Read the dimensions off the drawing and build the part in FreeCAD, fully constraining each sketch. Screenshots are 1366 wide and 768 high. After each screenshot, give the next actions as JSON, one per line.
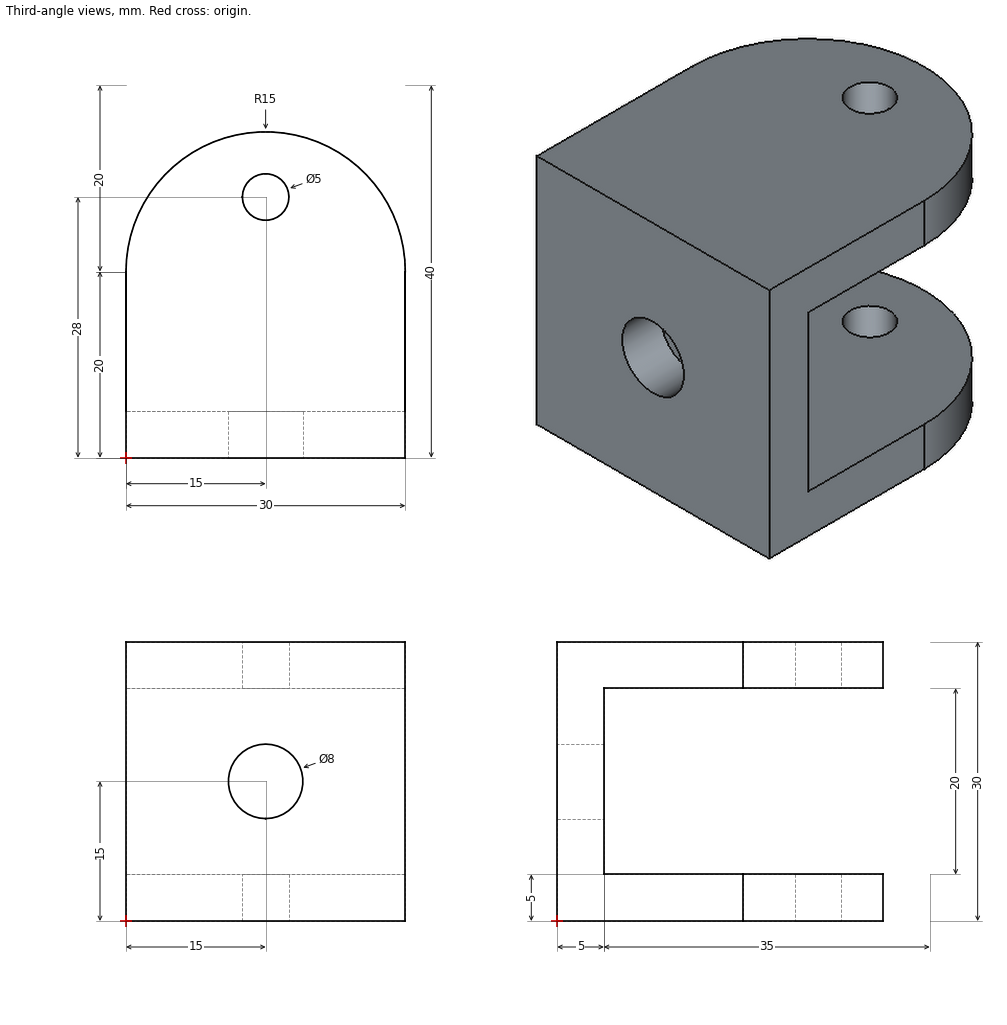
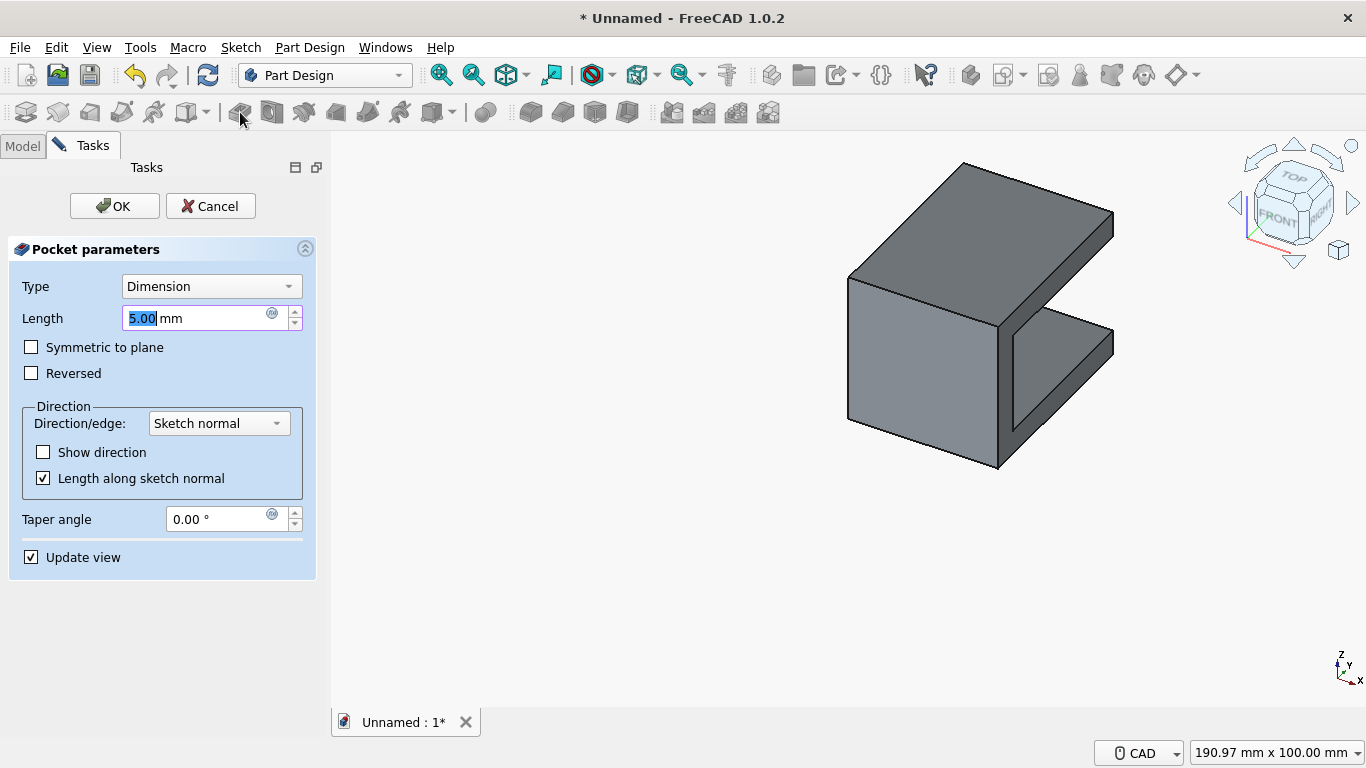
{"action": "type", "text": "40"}
{"action": "key", "text": "Tab"}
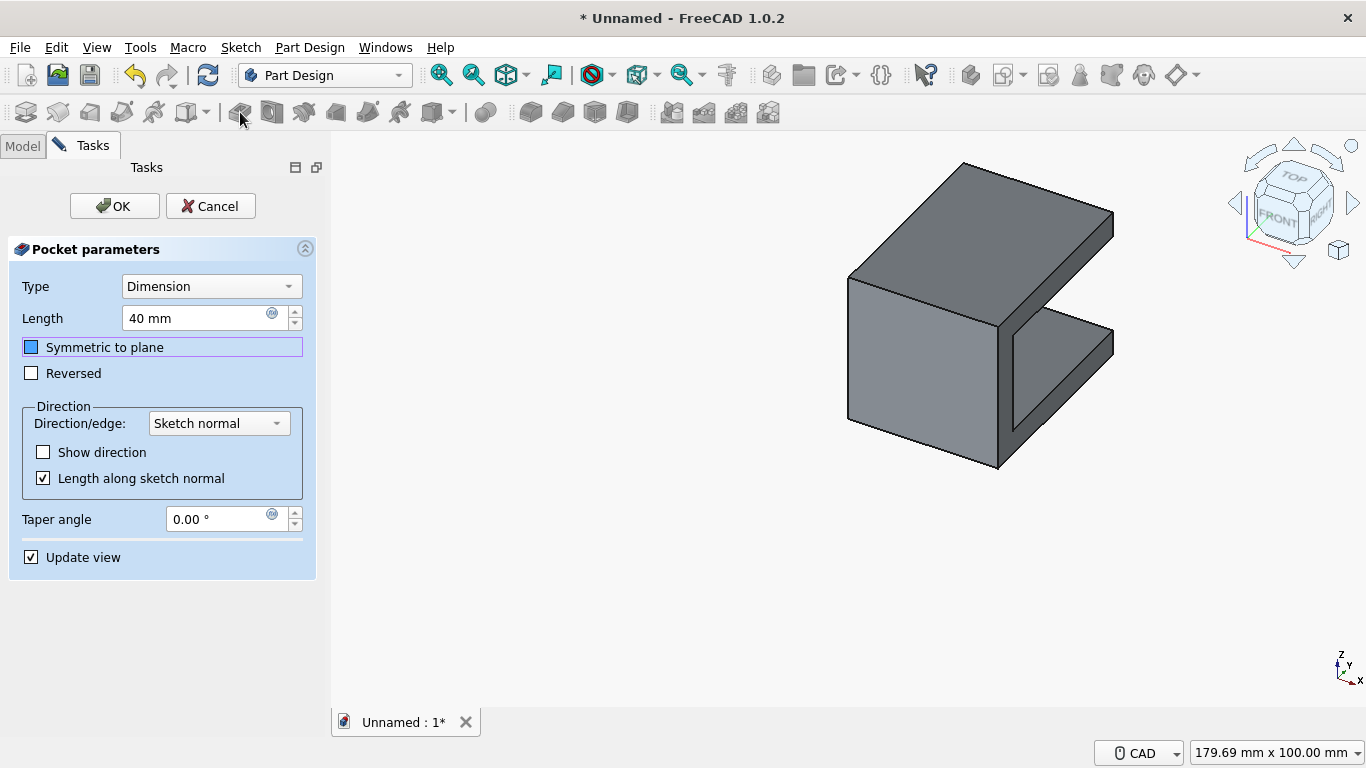
{"action": "left_click", "coordinate": [30, 373]}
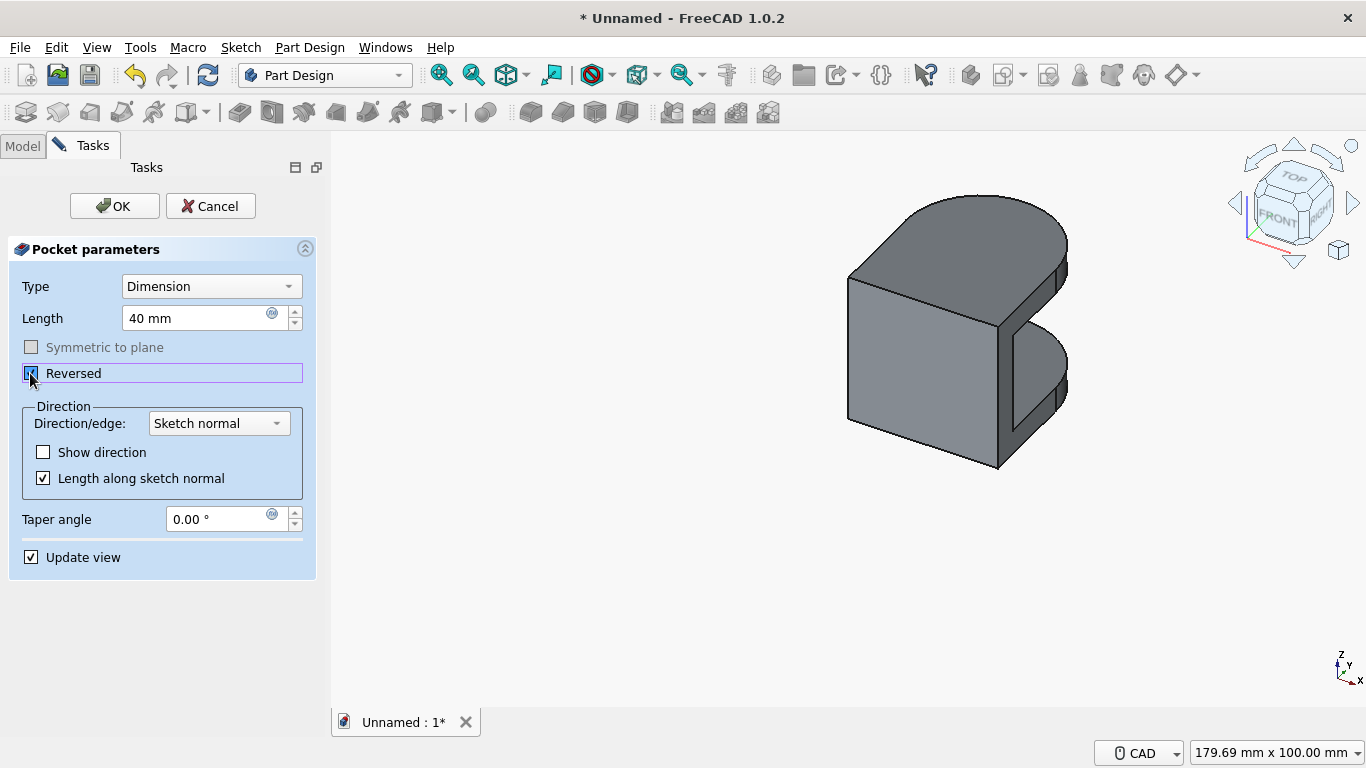
{"action": "left_click", "coordinate": [115, 206]}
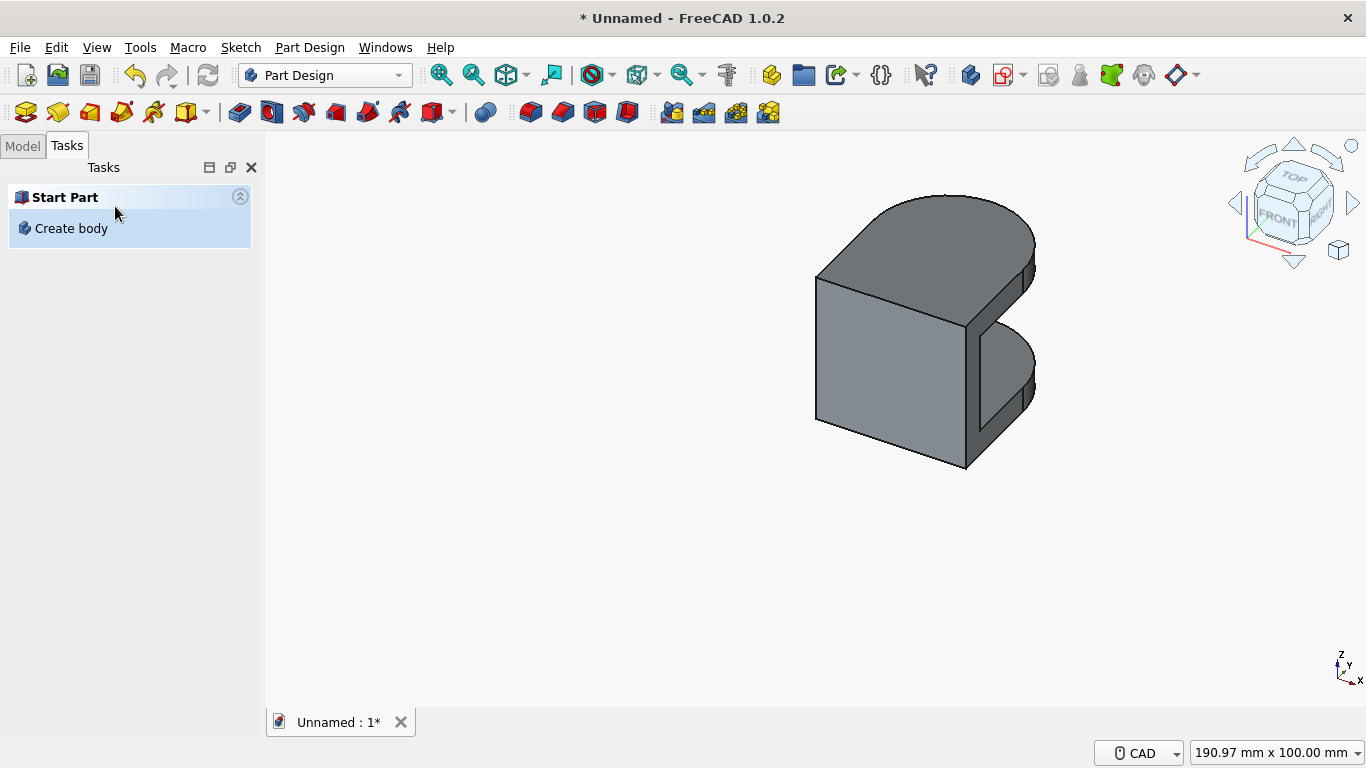
{"action": "key", "text": "5"}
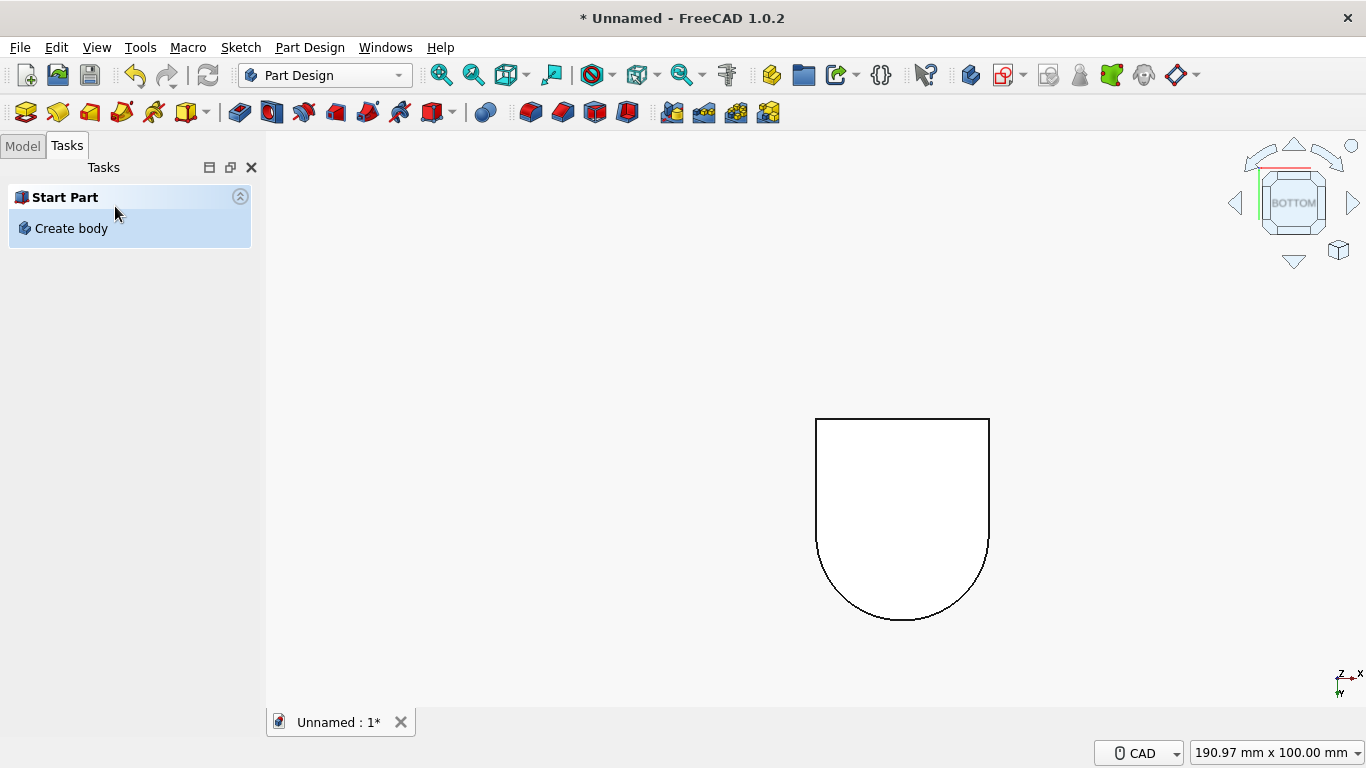
{"action": "left_click", "coordinate": [442, 76]}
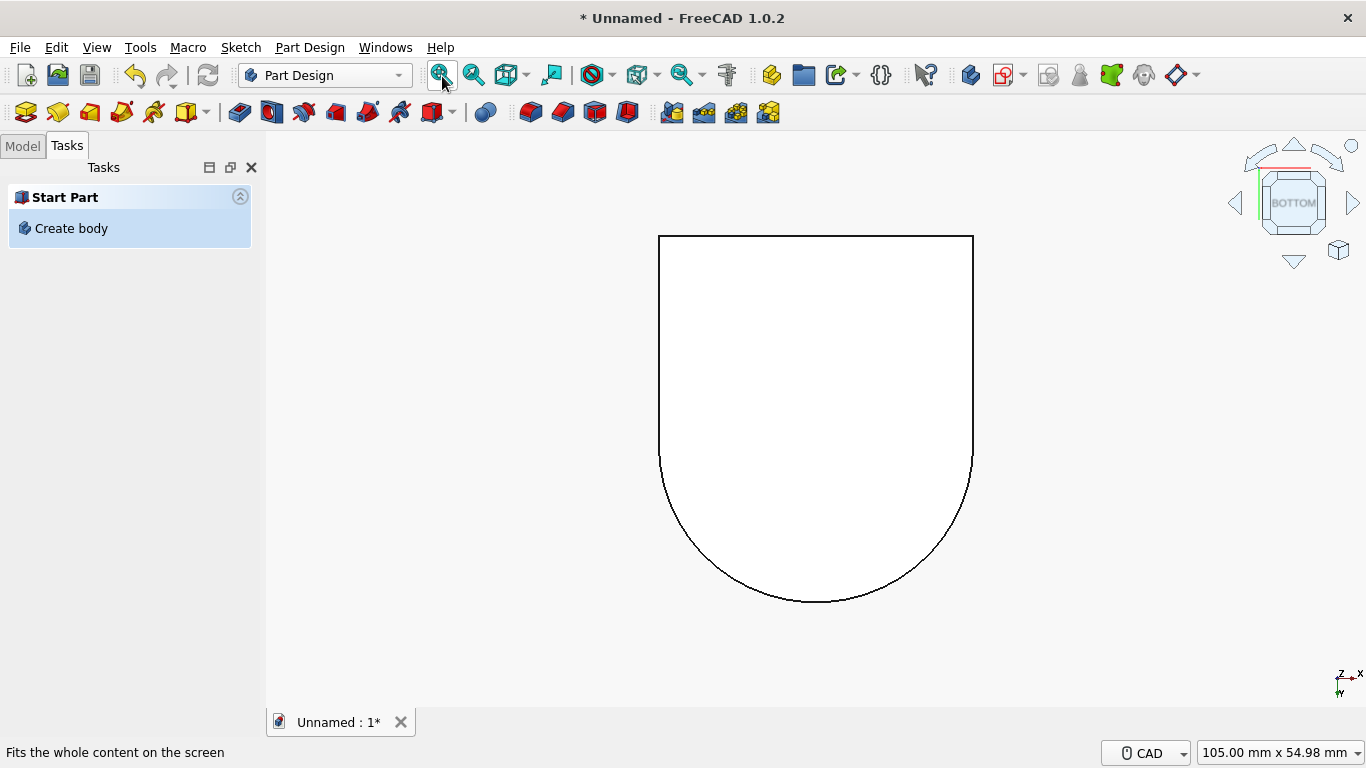
{"action": "left_click", "coordinate": [816, 418]}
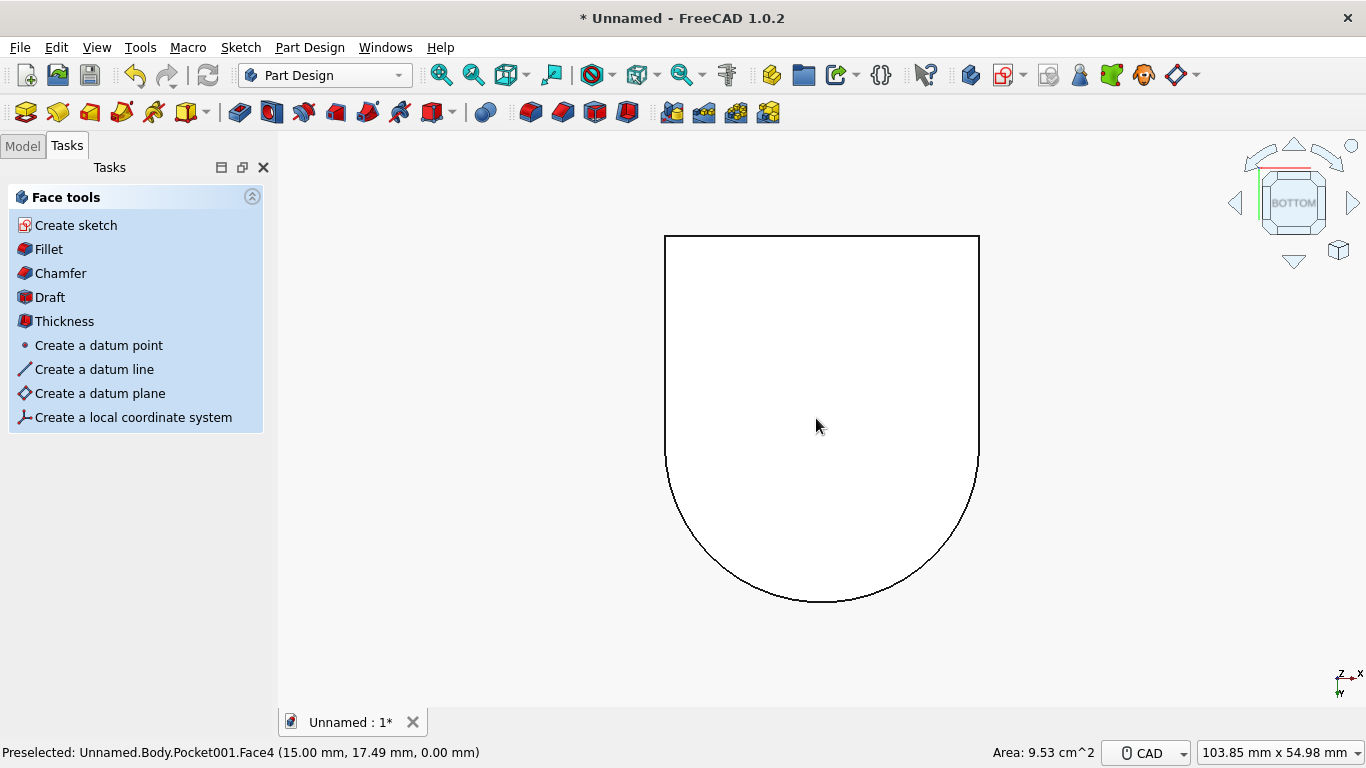
{"action": "left_click", "coordinate": [1004, 76]}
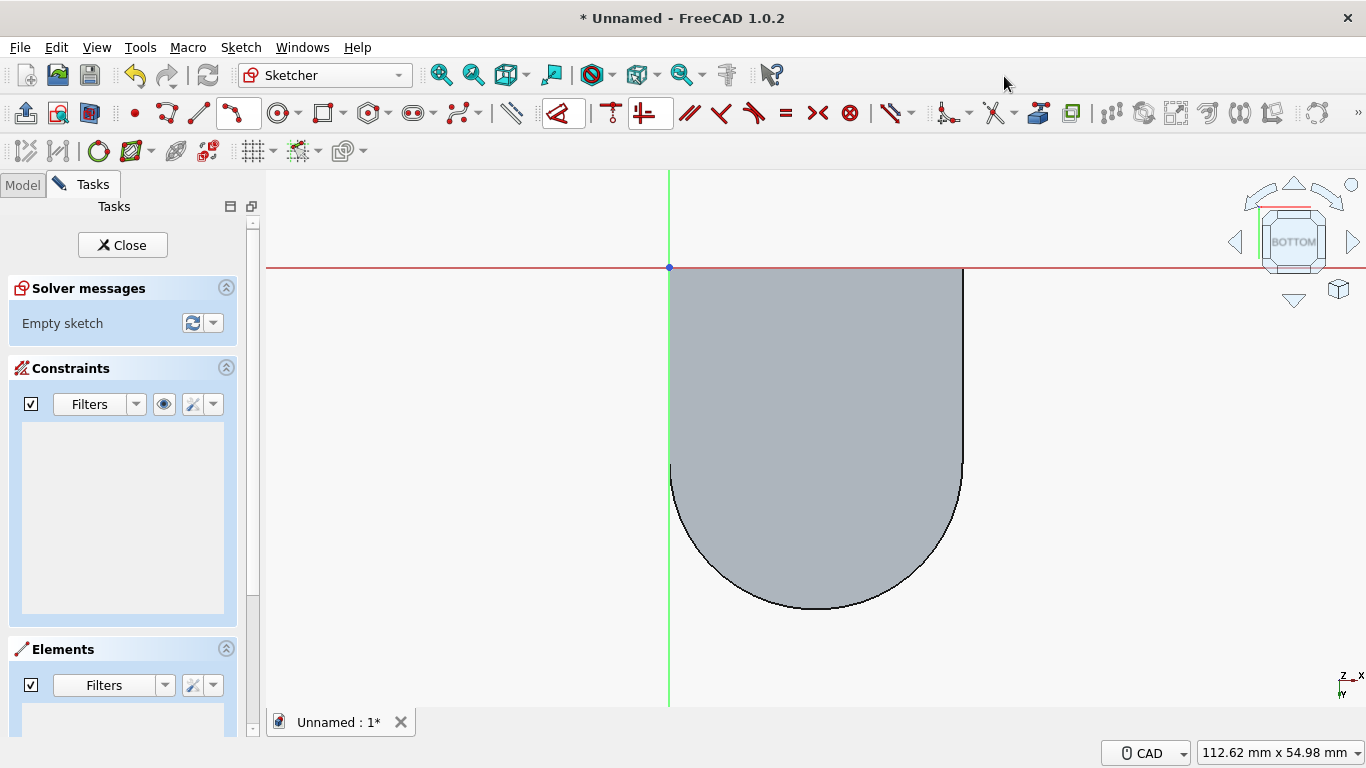
{"action": "scroll", "coordinate": [827, 557], "scroll_direction": "up", "scroll_amount": 10}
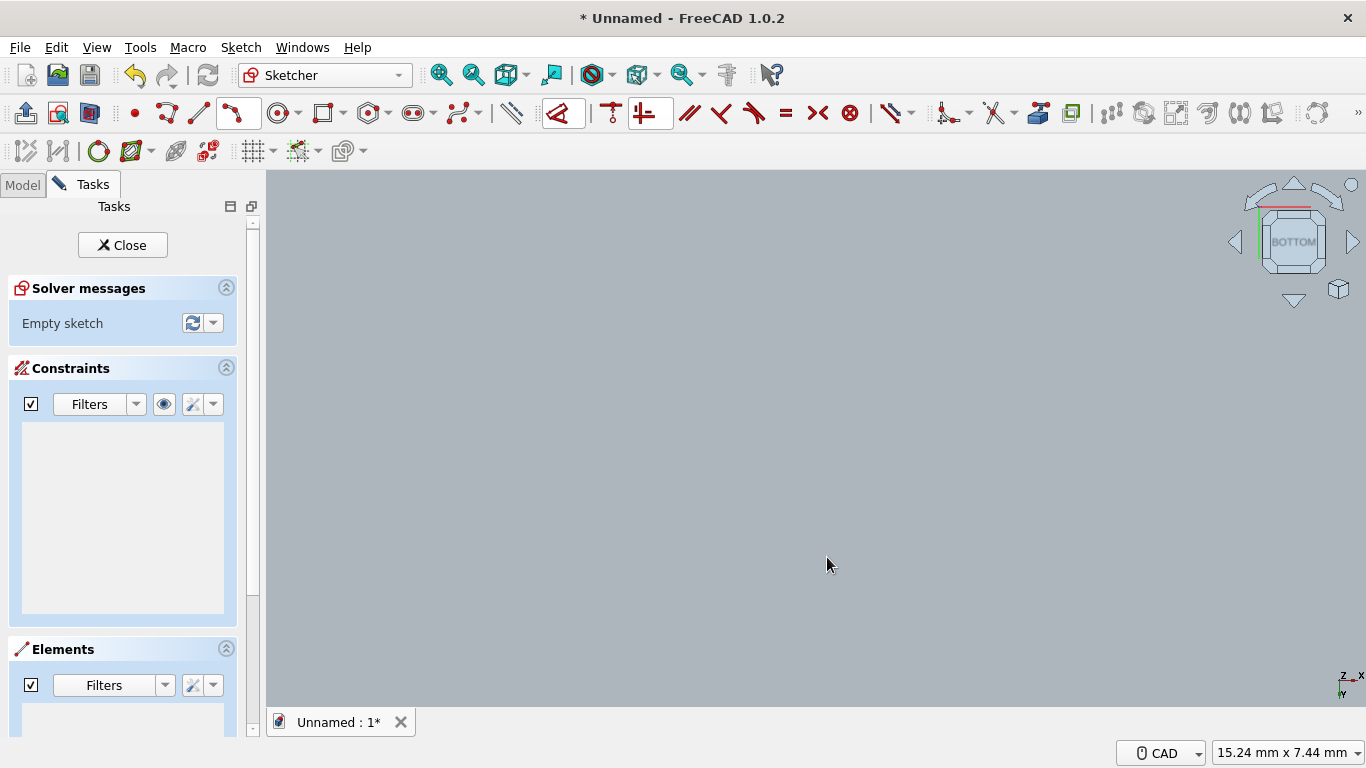
{"action": "left_click", "coordinate": [278, 114]}